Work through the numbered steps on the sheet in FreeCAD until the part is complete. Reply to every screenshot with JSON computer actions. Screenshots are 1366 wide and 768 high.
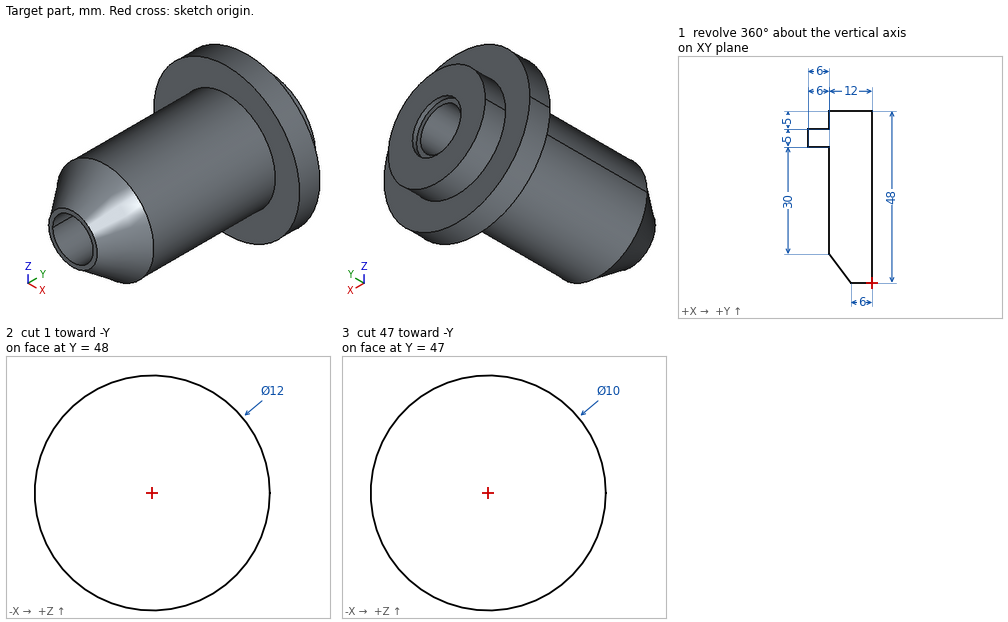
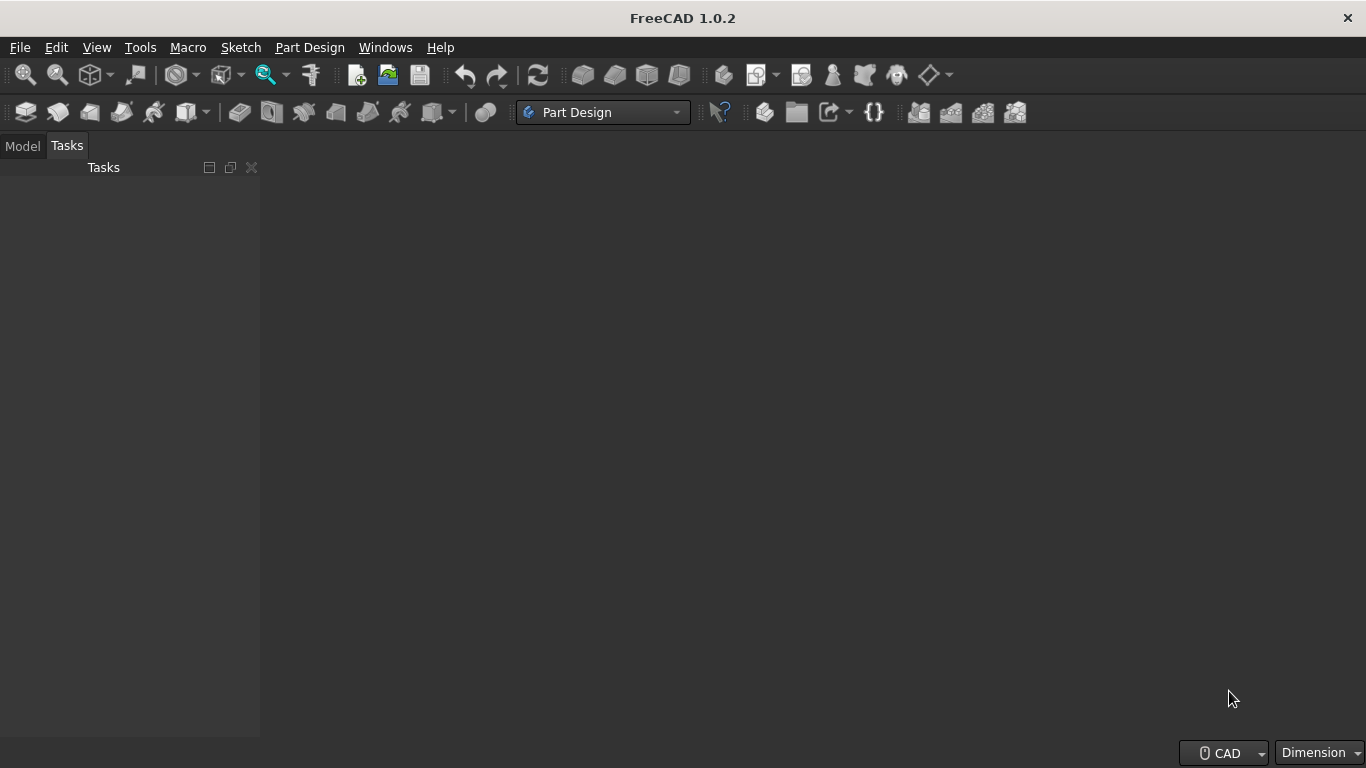
{"action": "left_click", "coordinate": [356, 76]}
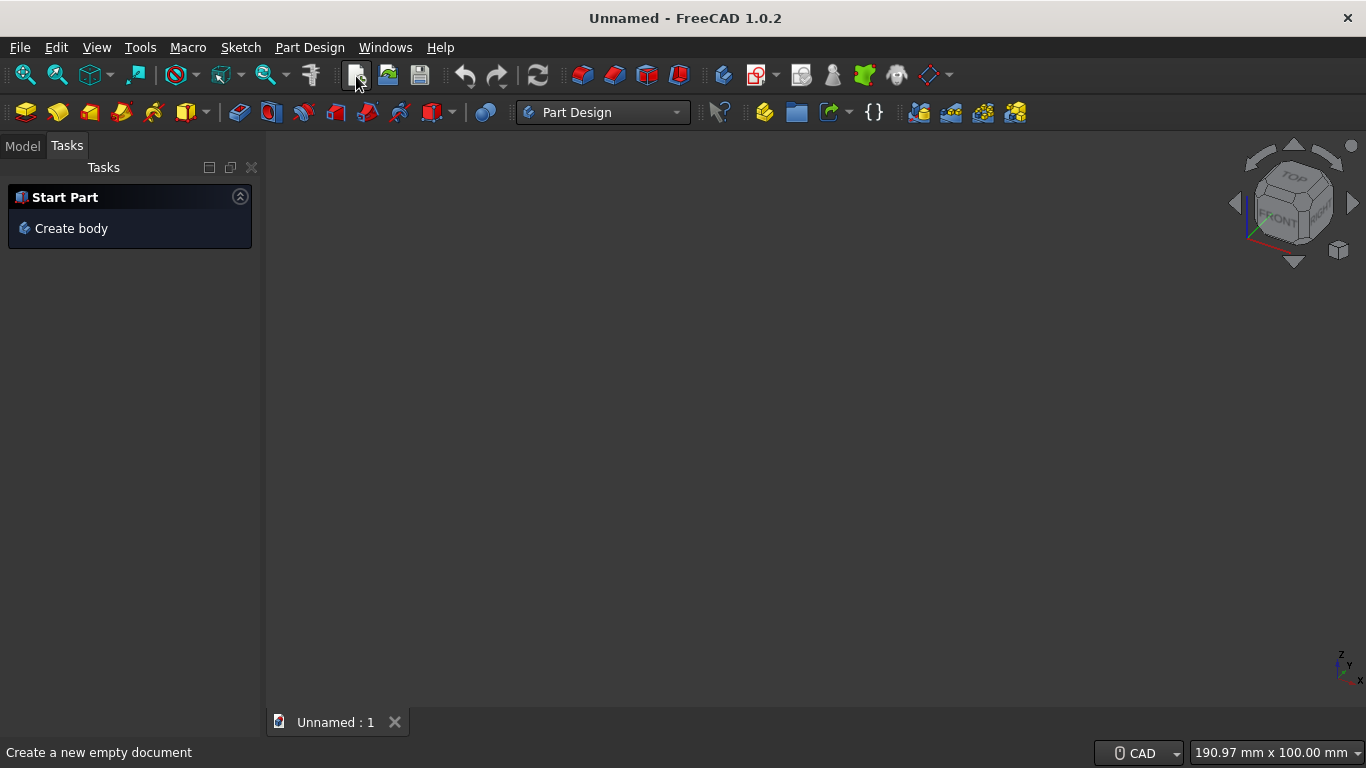
{"action": "left_click", "coordinate": [756, 76]}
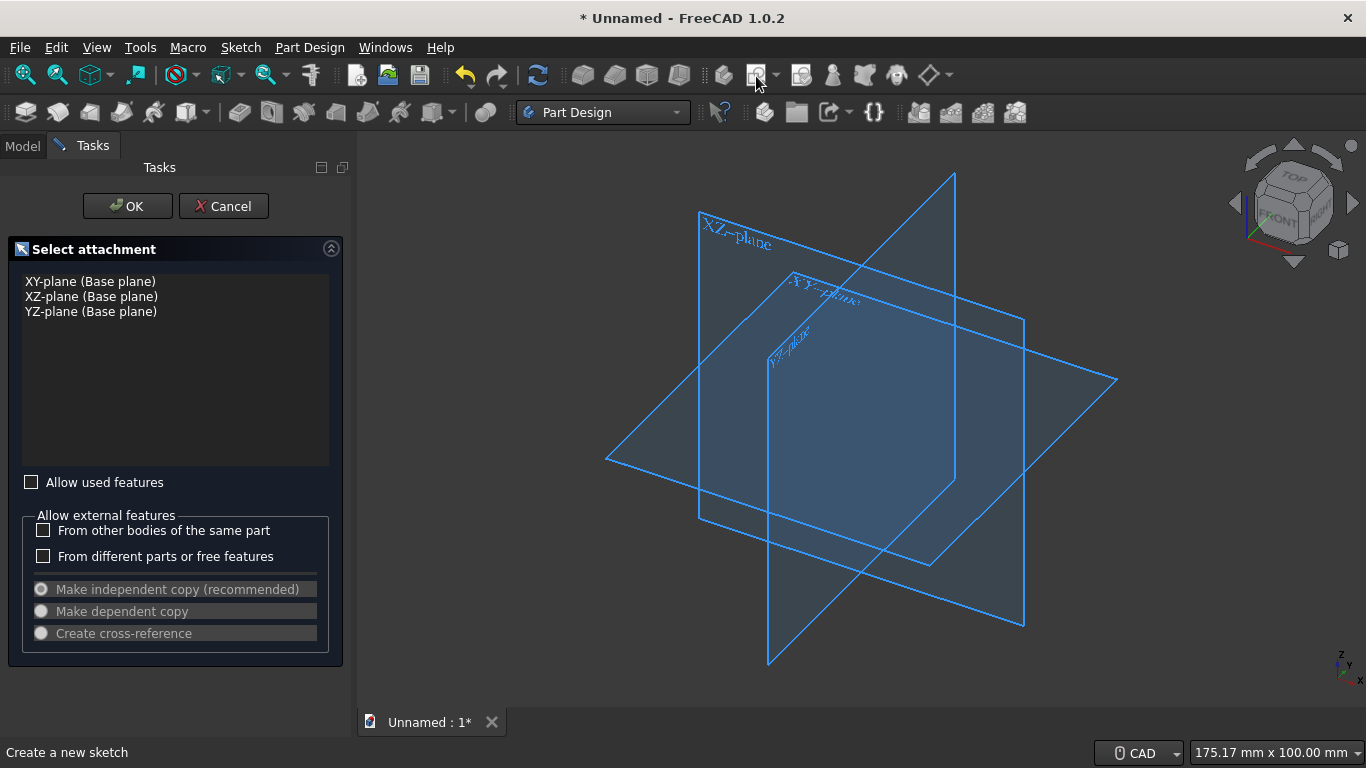
{"action": "left_click", "coordinate": [82, 282]}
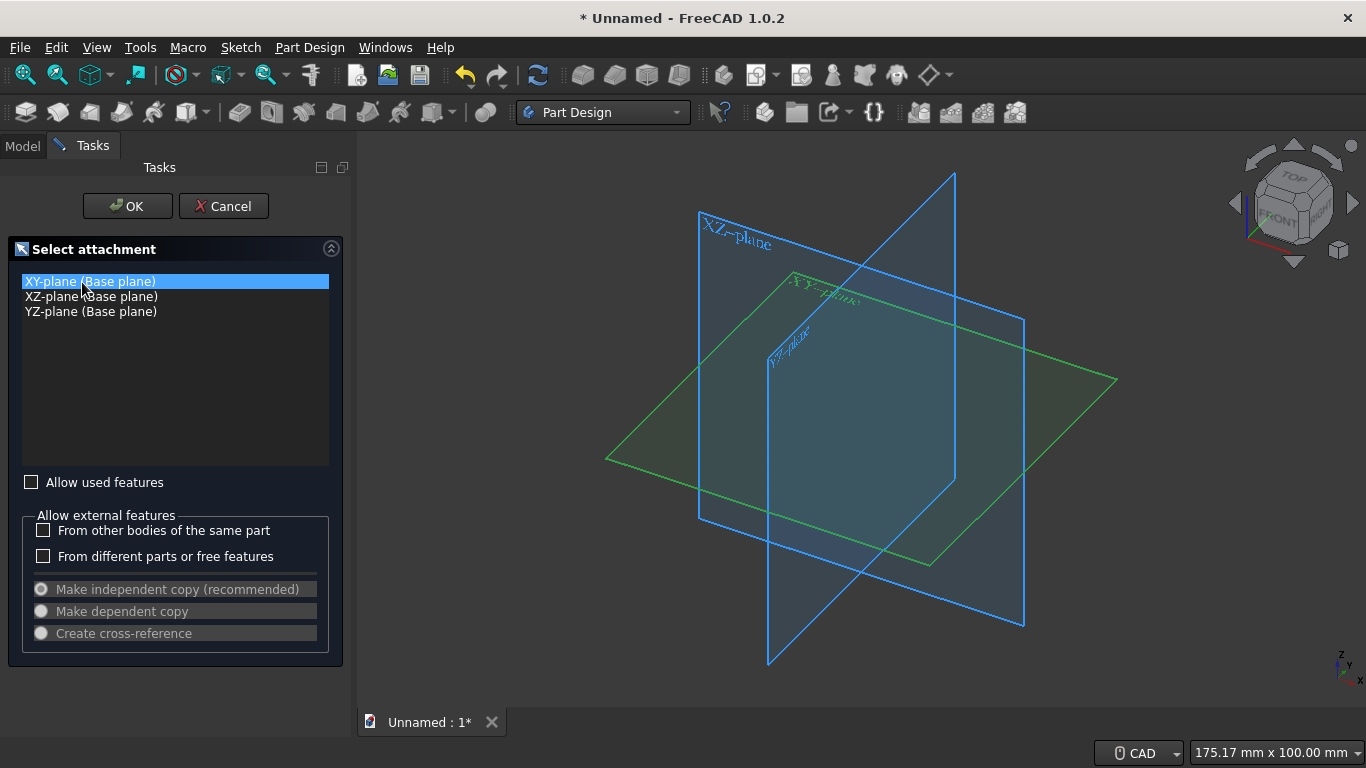
{"action": "left_click", "coordinate": [128, 206]}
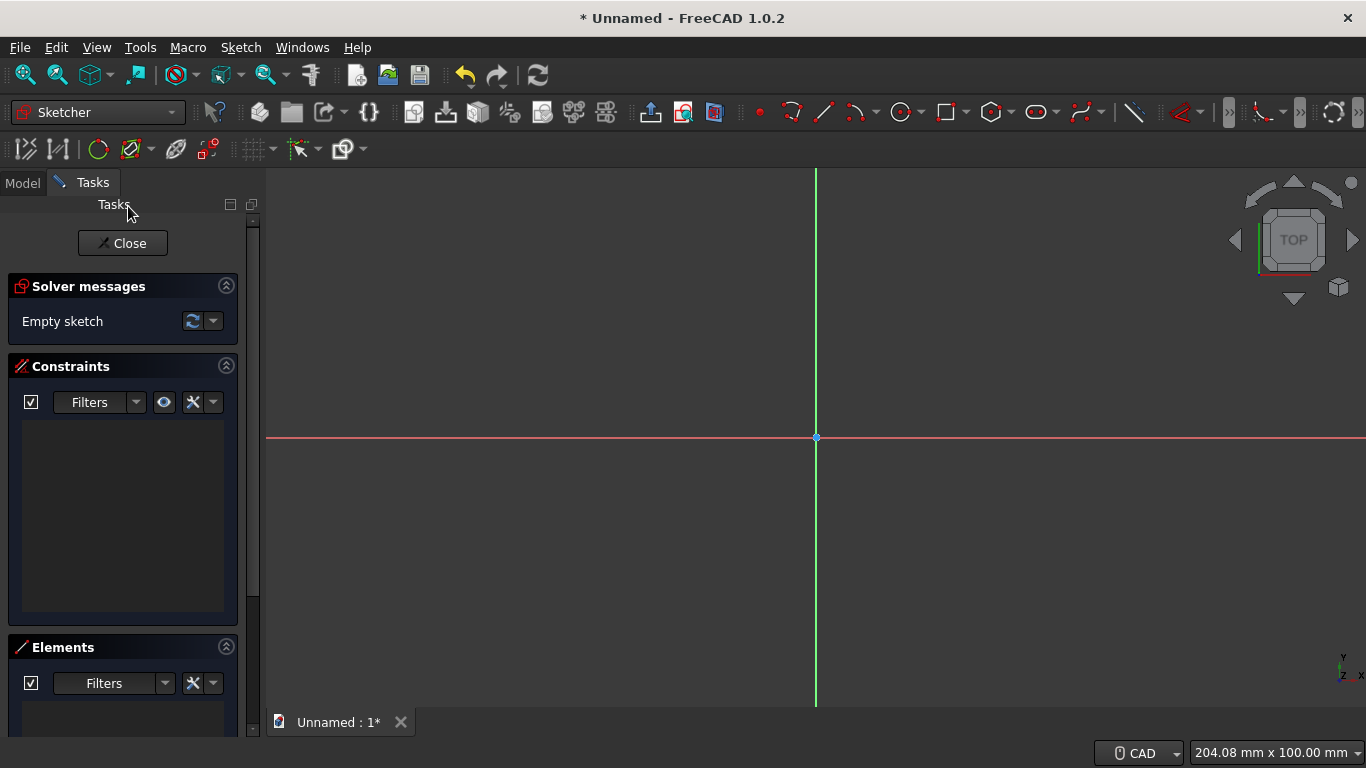
{"action": "scroll", "coordinate": [657, 679], "scroll_direction": "down", "scroll_amount": 1}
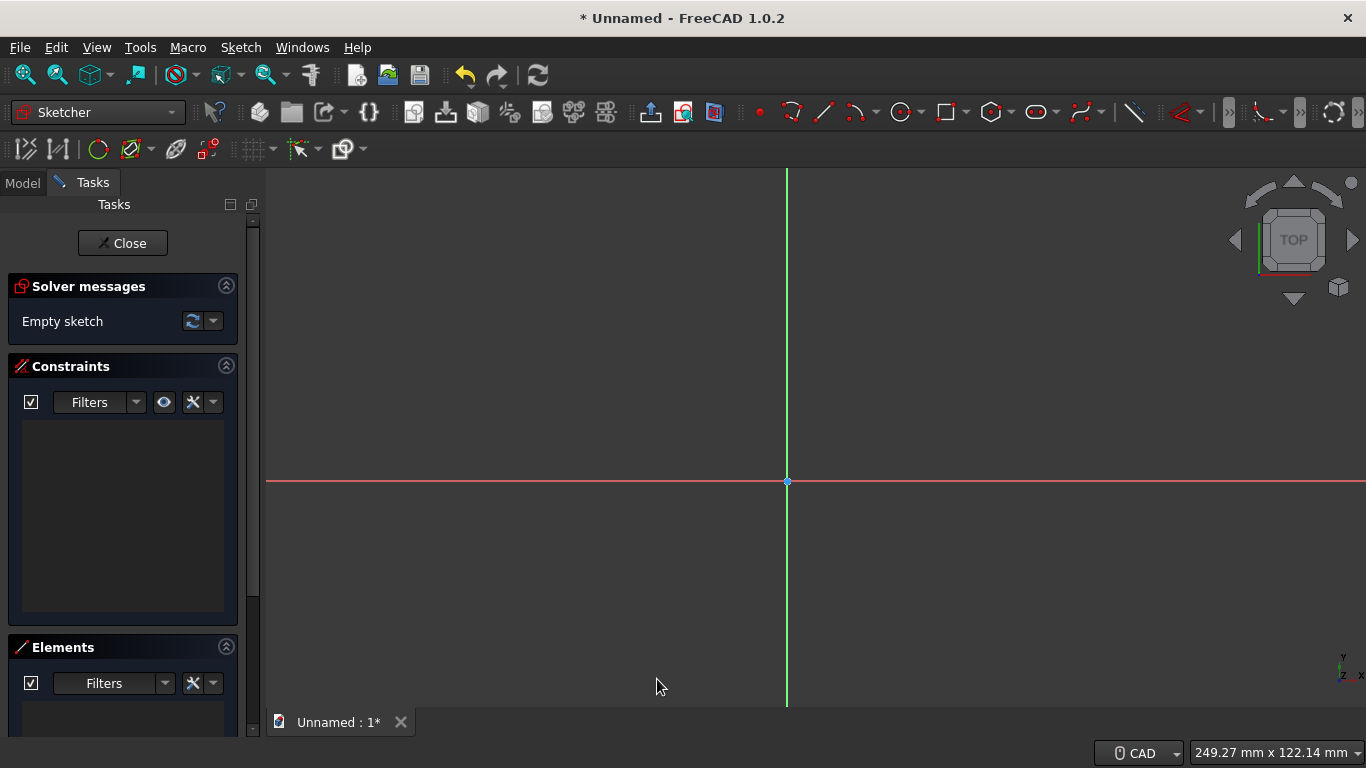
{"action": "scroll", "coordinate": [748, 250], "scroll_direction": "up", "scroll_amount": 2}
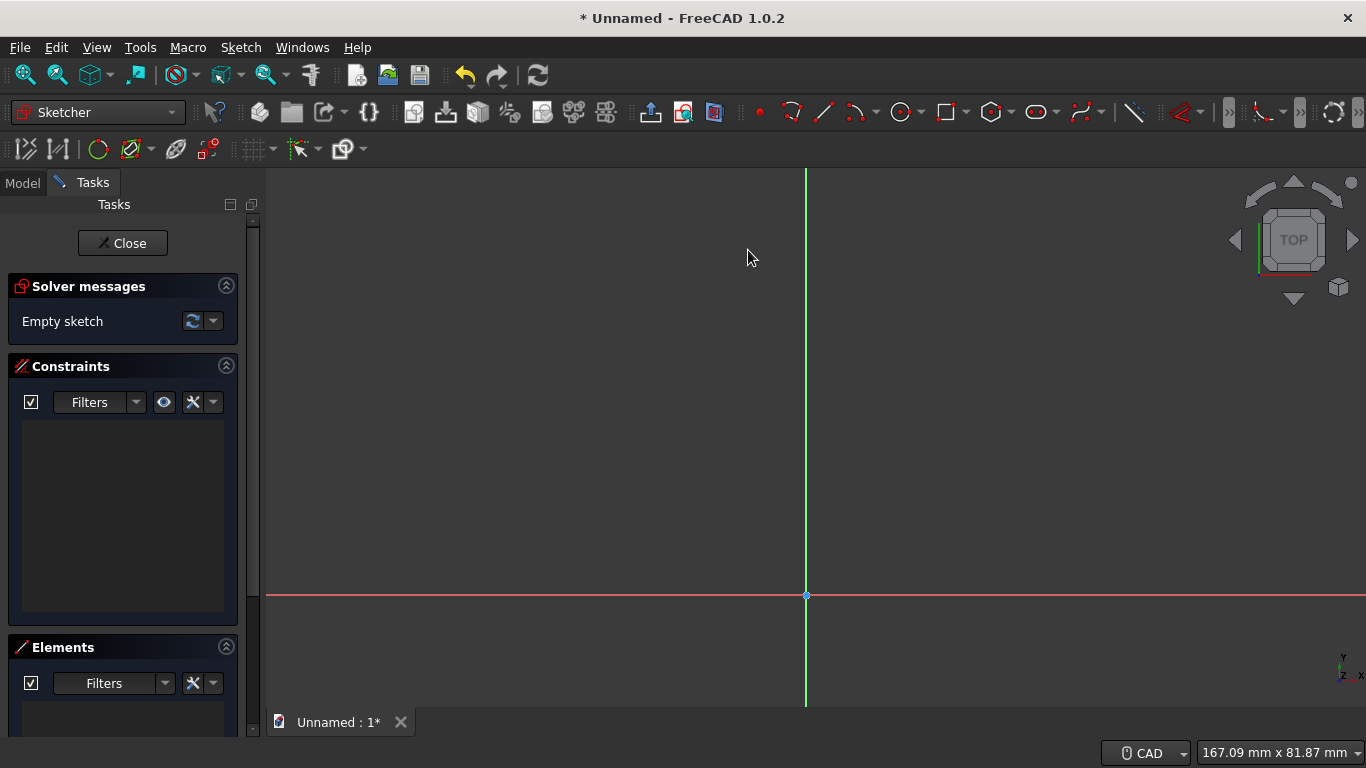
{"action": "left_click", "coordinate": [792, 112]}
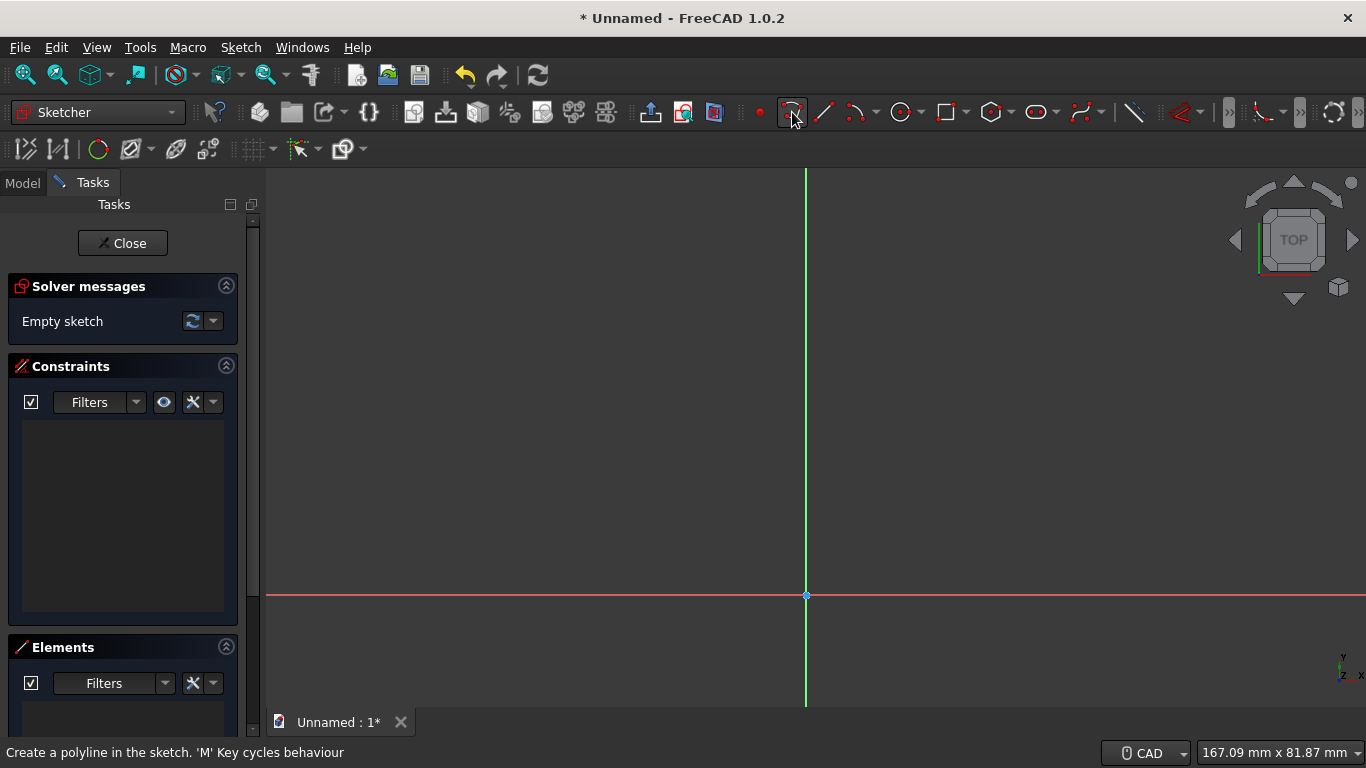
{"action": "left_click", "coordinate": [806, 595]}
{"action": "left_click", "coordinate": [797, 279]}
{"action": "left_click", "coordinate": [727, 279]}
{"action": "left_click", "coordinate": [727, 312]}
{"action": "left_click", "coordinate": [688, 312]}
{"action": "left_click", "coordinate": [688, 345]}
{"action": "left_click", "coordinate": [727, 345]}
{"action": "left_click", "coordinate": [727, 543]}
{"action": "left_click", "coordinate": [767, 586]}
{"action": "left_click", "coordinate": [806, 595]}
{"action": "key", "text": "Escape"}
{"action": "key", "text": "Escape"}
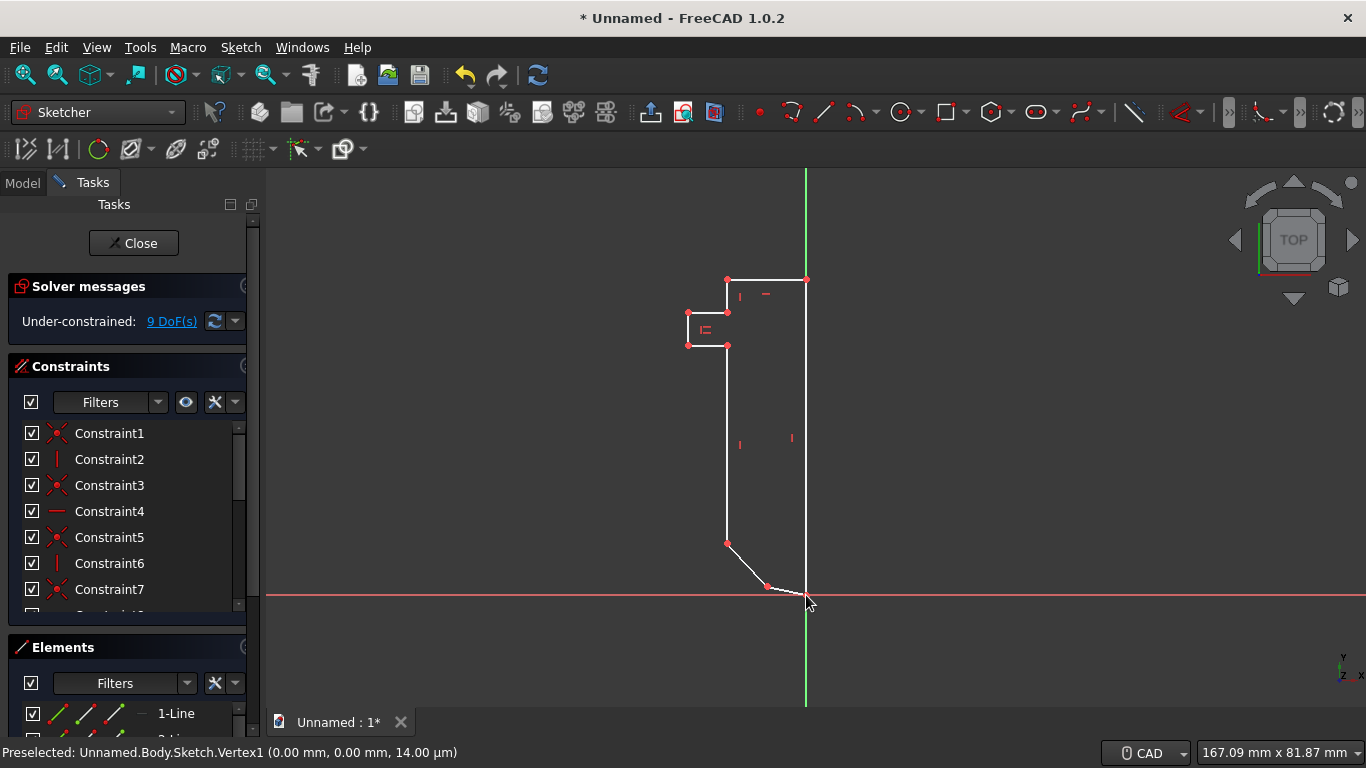
{"action": "left_click", "coordinate": [795, 593]}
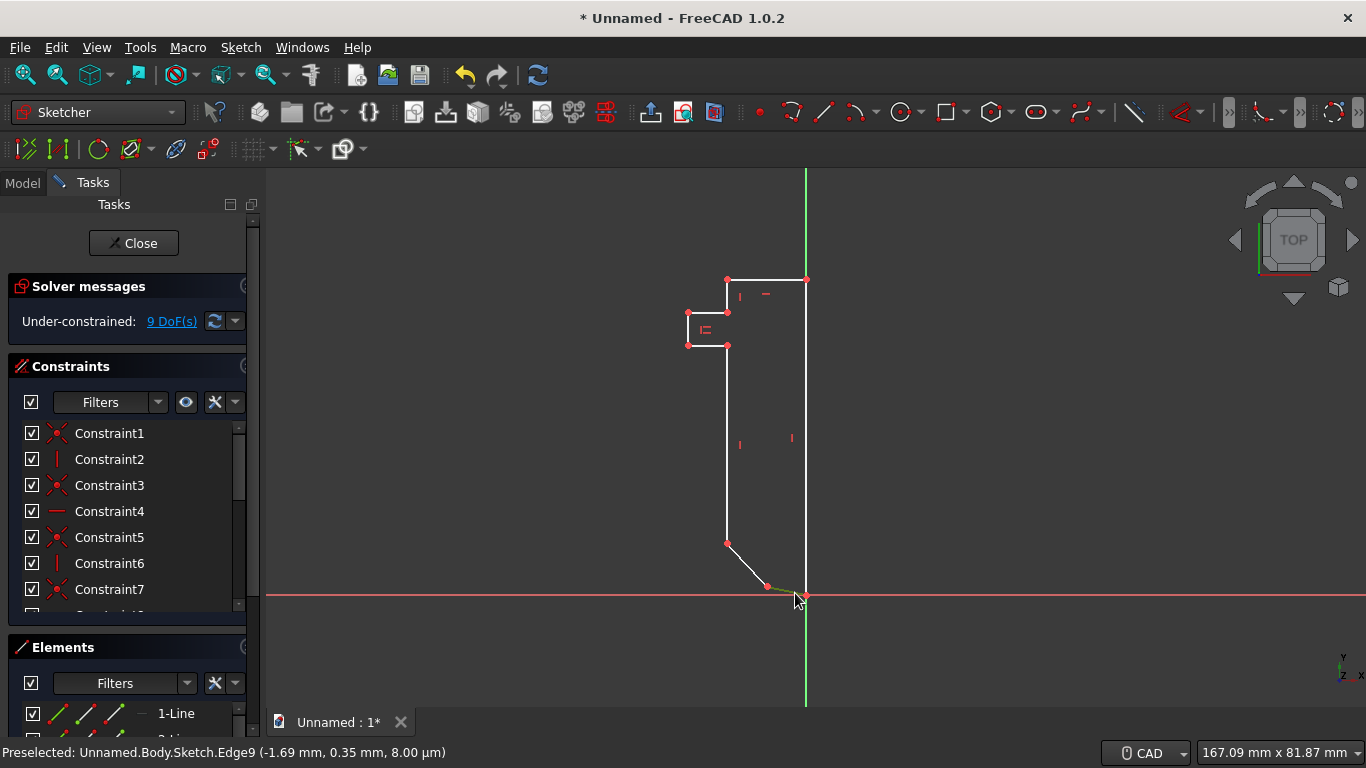
{"action": "key", "text": "h"}